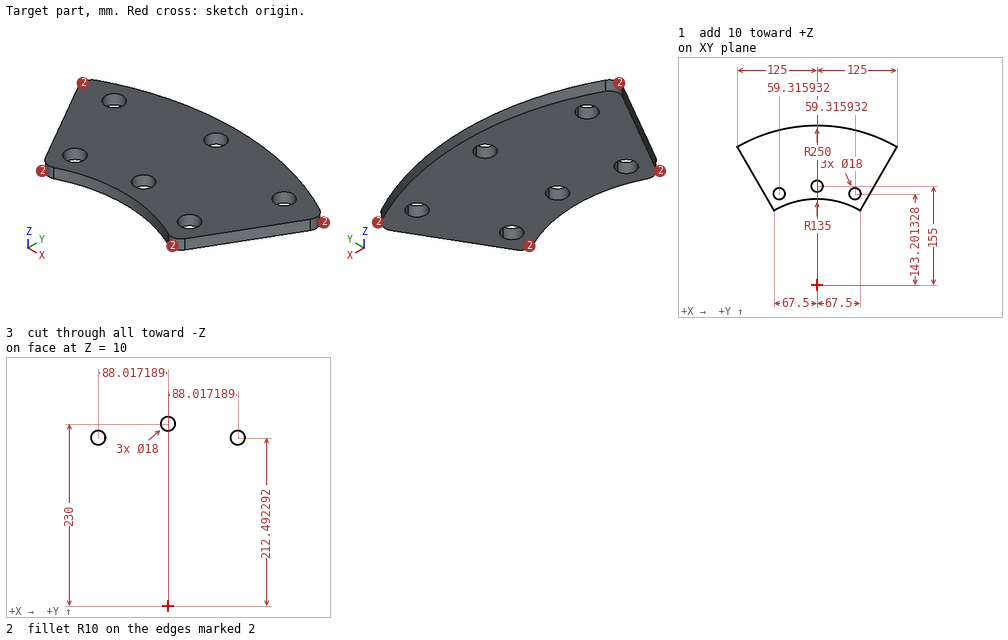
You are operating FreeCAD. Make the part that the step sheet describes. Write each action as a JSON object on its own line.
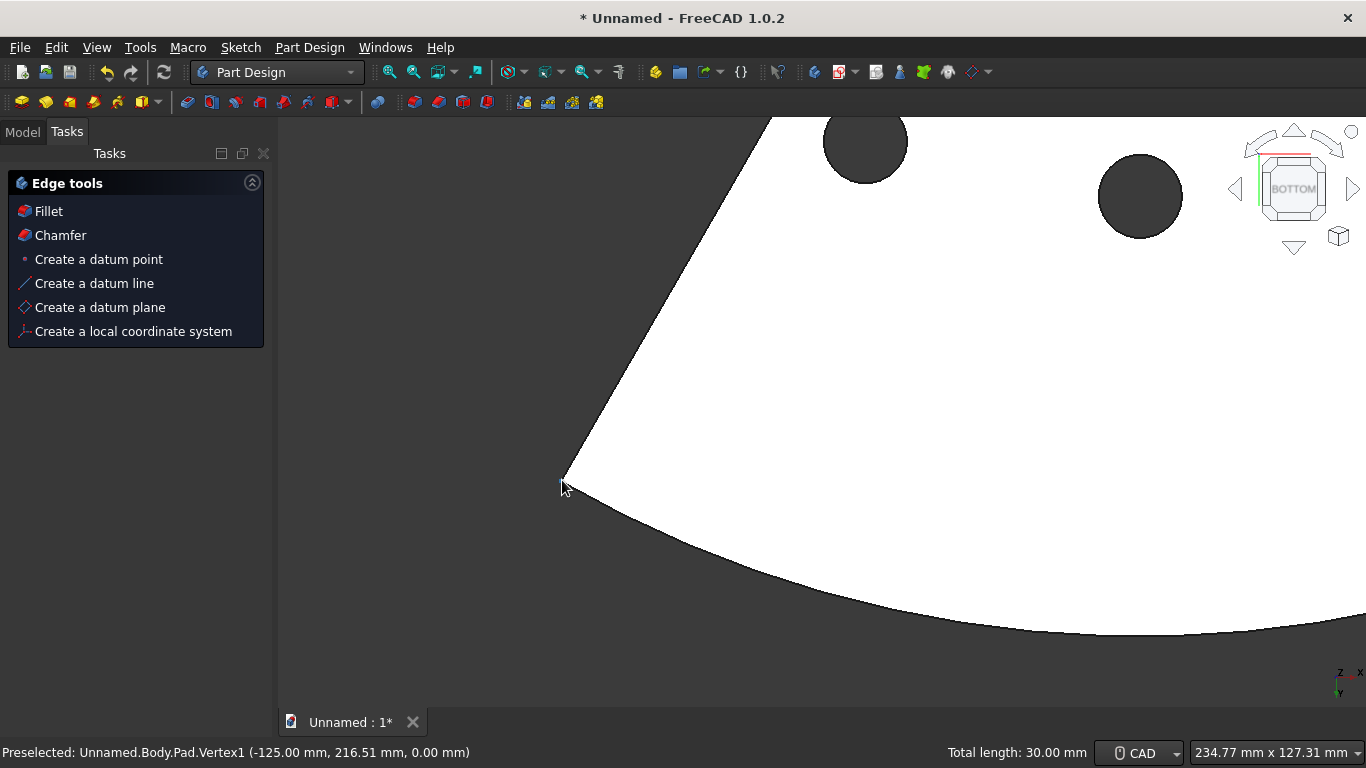
{"action": "left_click", "coordinate": [390, 72]}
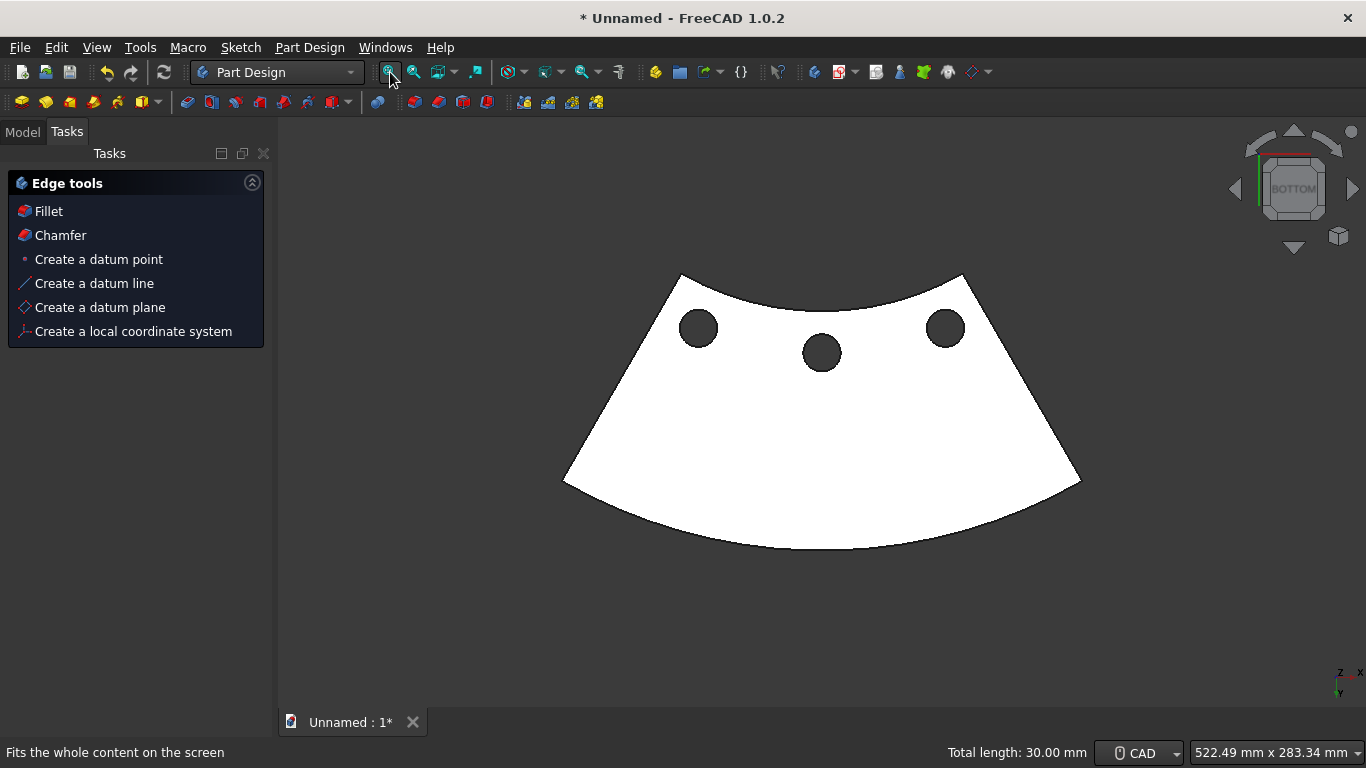
{"action": "key", "text": "4"}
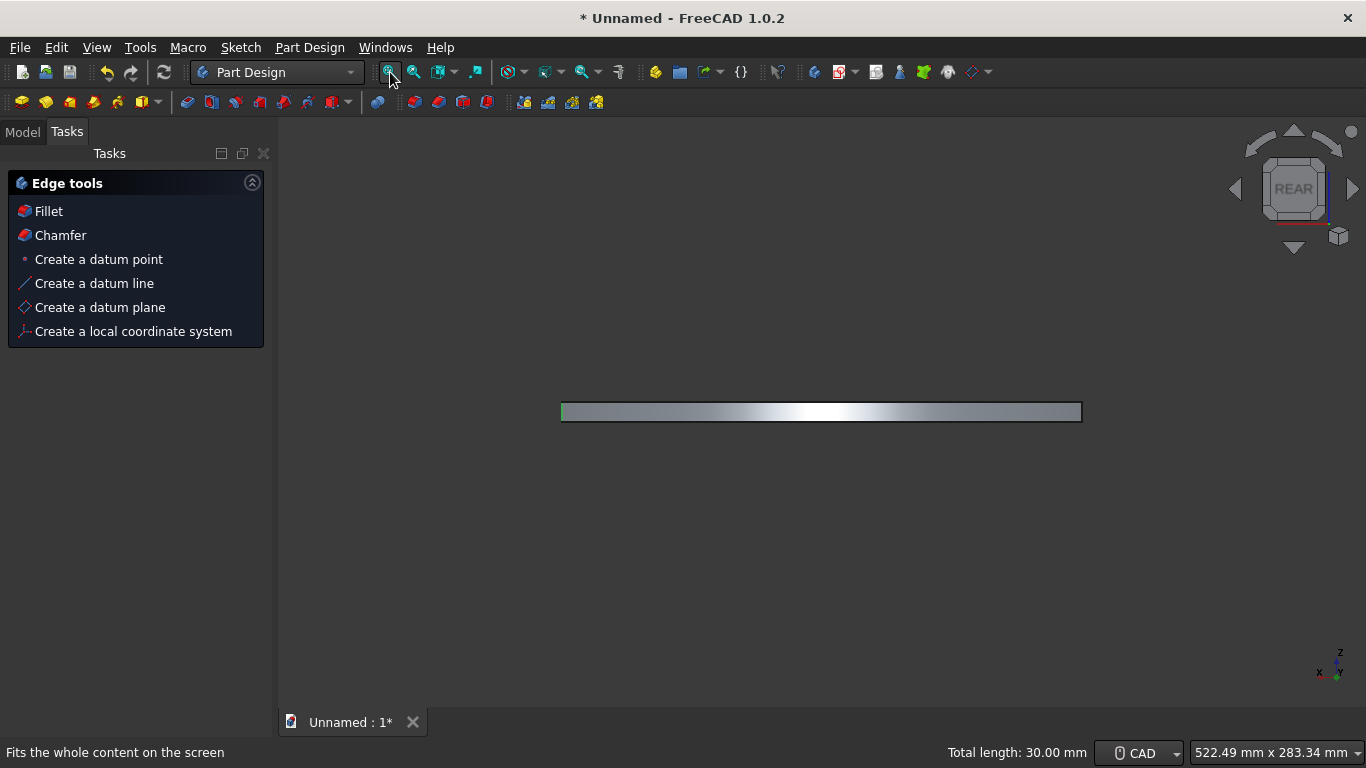
{"action": "scroll", "coordinate": [1082, 411], "scroll_direction": "up", "scroll_amount": 4}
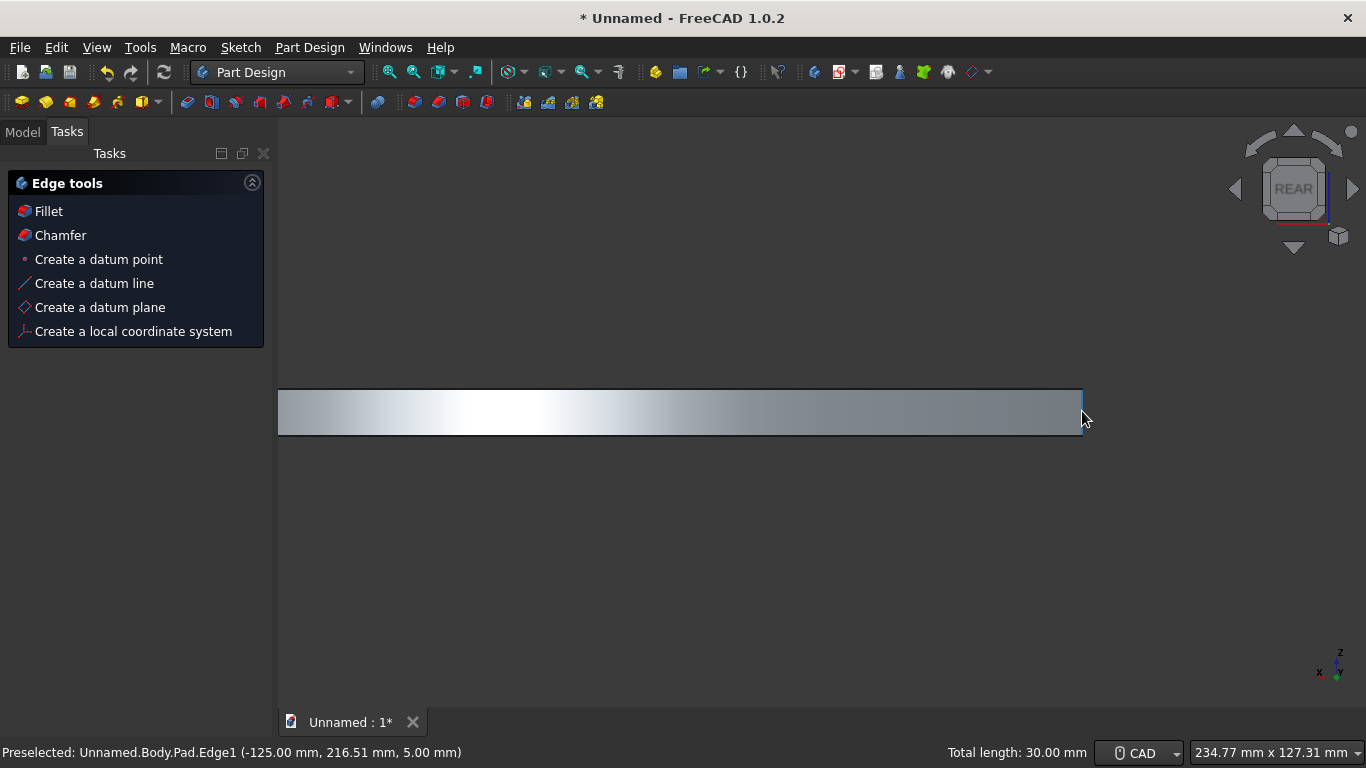
{"action": "key", "text": "v f"}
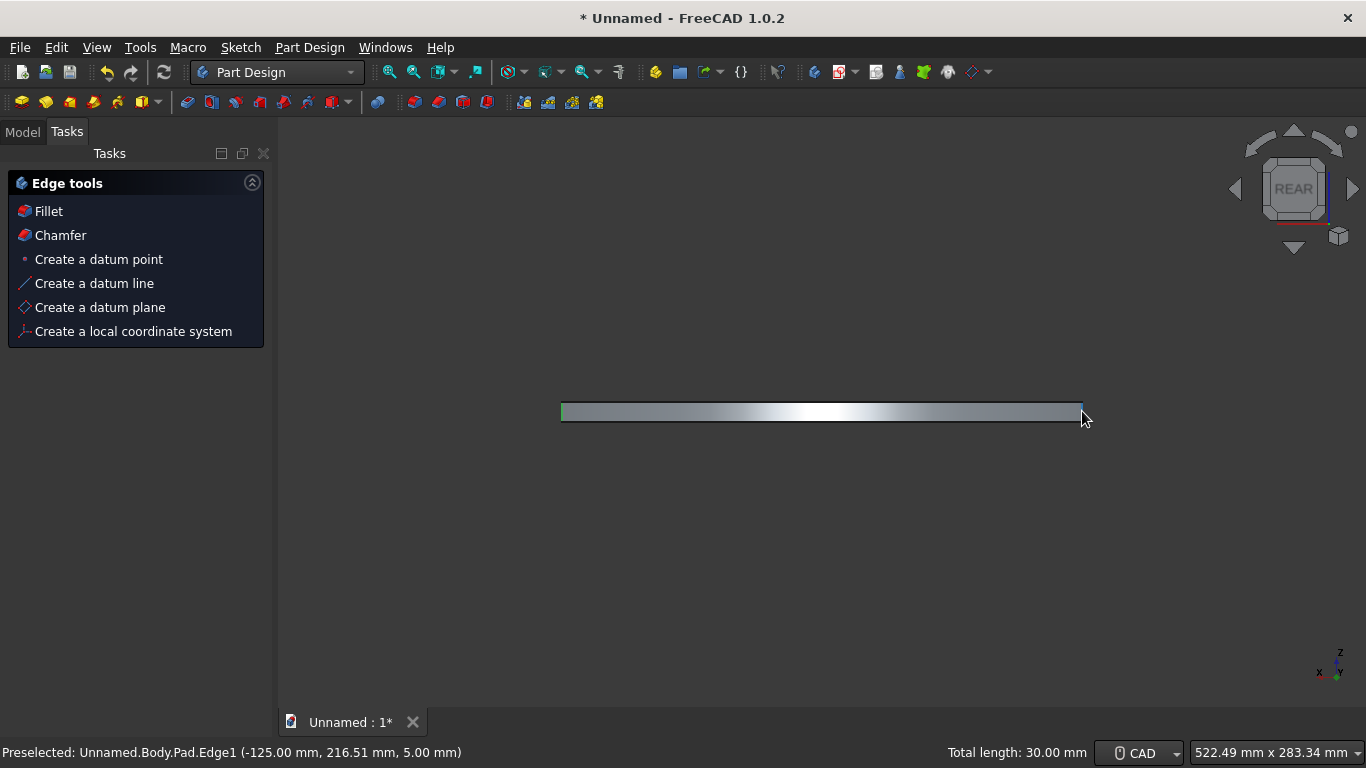
{"action": "key", "text": "6"}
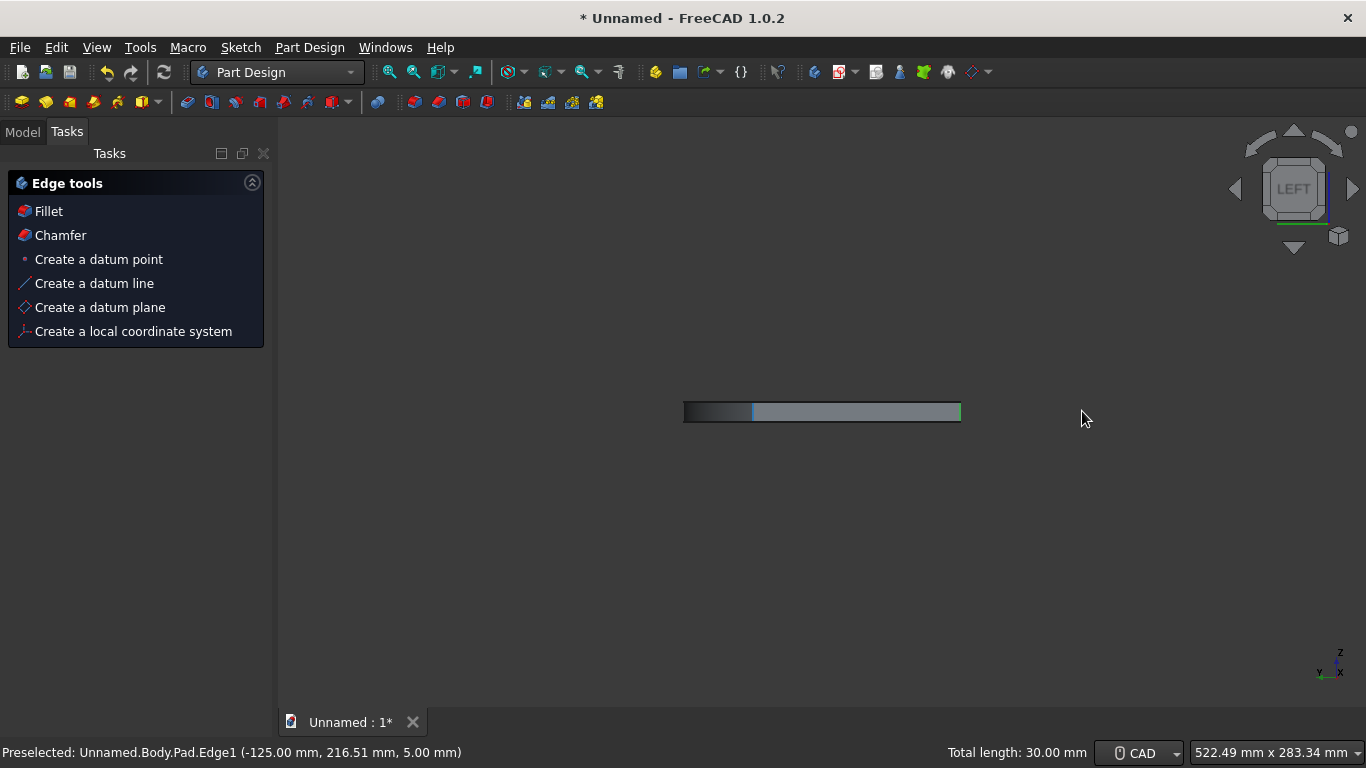
{"action": "left_click", "coordinate": [390, 72]}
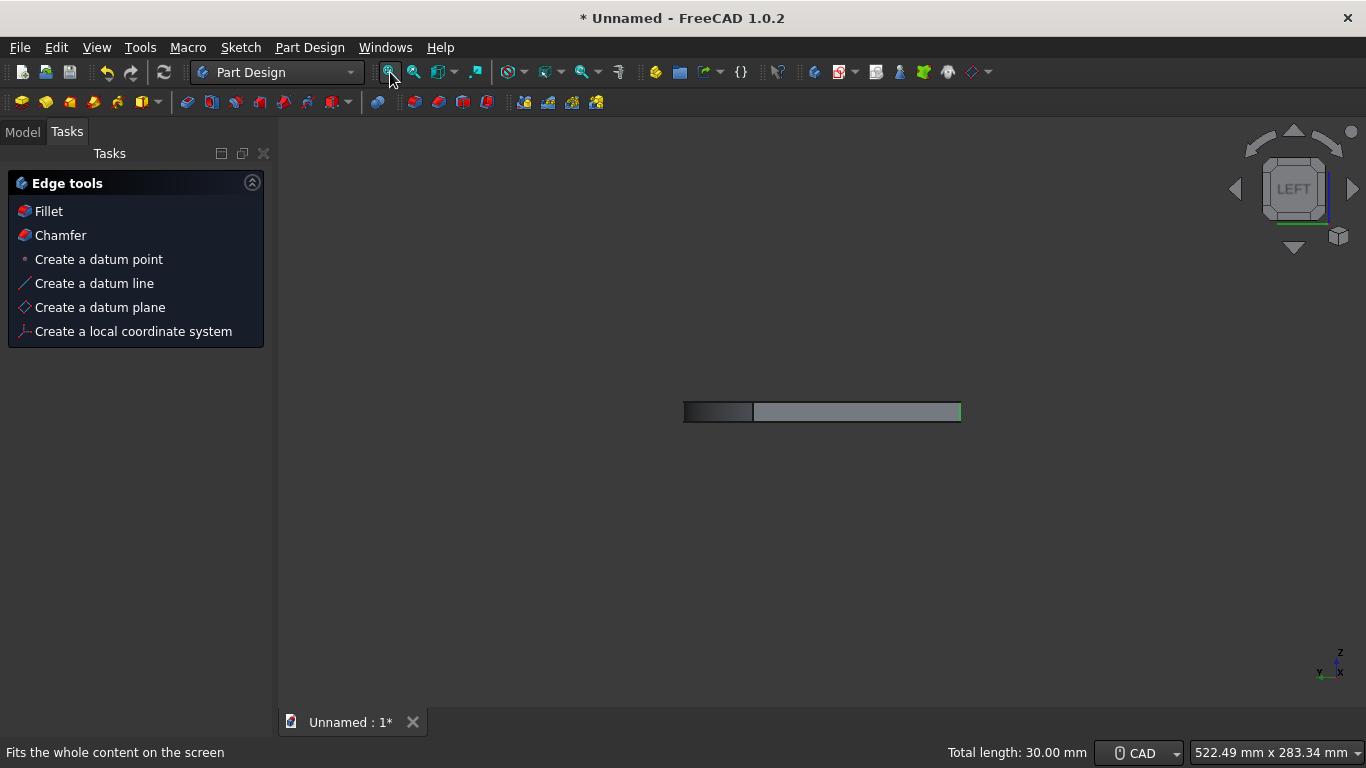
{"action": "left_click", "coordinate": [753, 411], "text": "ctrl"}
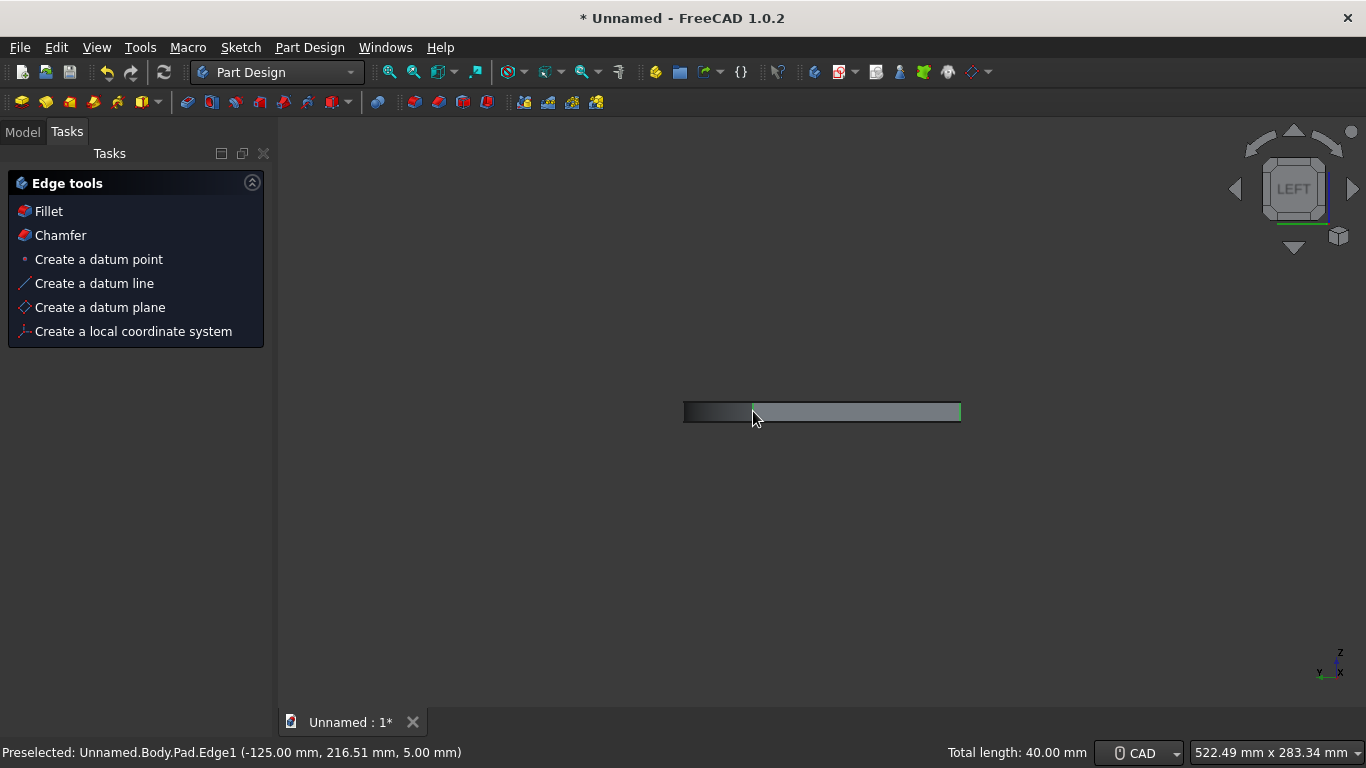
{"action": "left_click", "coordinate": [416, 102]}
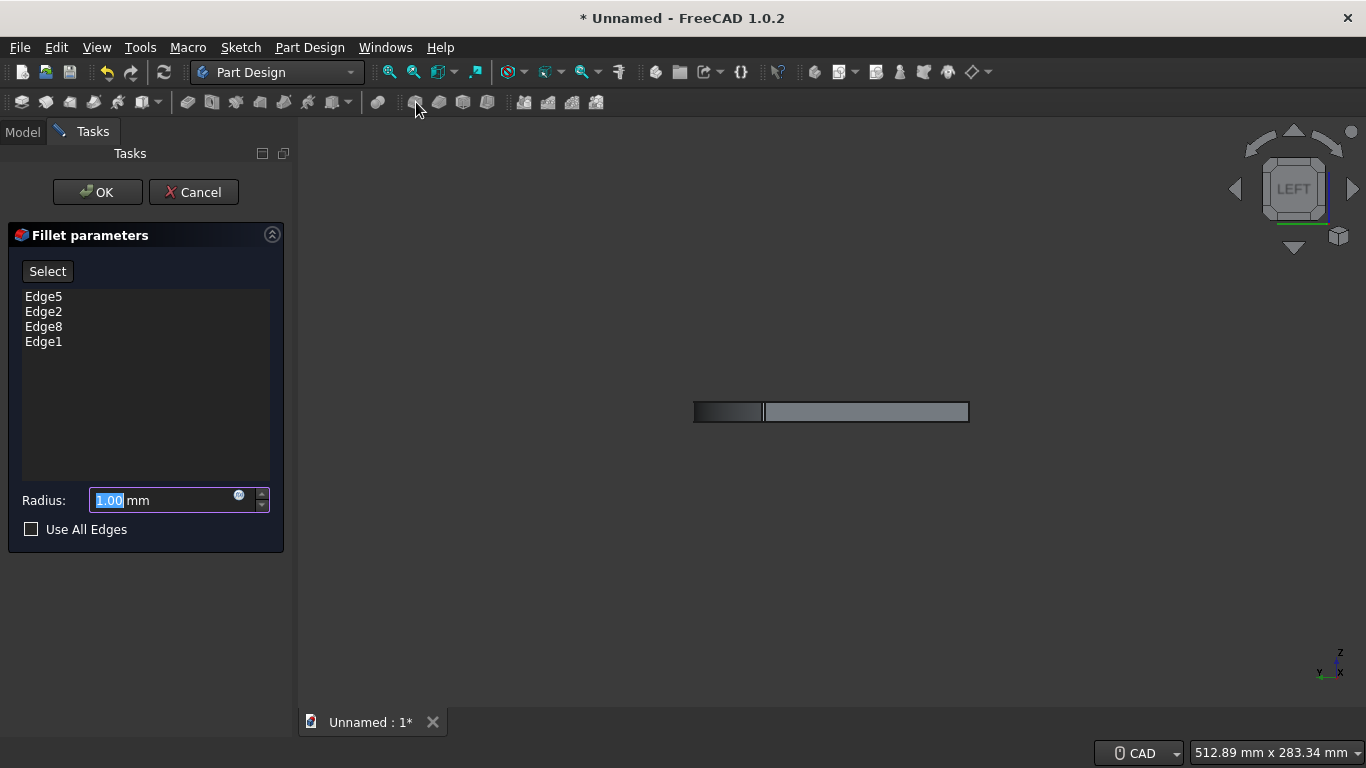
{"action": "type", "text": "10"}
{"action": "key", "text": "Tab"}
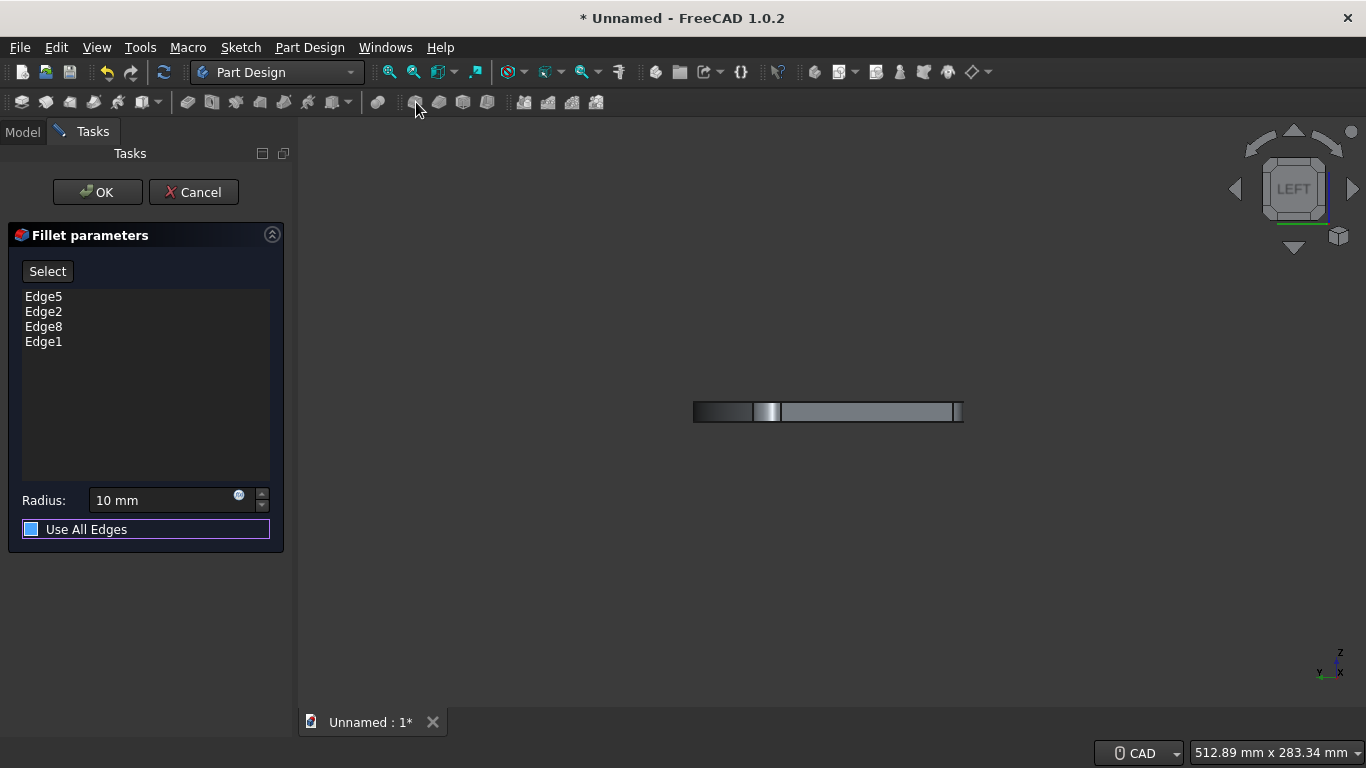
{"action": "left_click", "coordinate": [98, 192]}